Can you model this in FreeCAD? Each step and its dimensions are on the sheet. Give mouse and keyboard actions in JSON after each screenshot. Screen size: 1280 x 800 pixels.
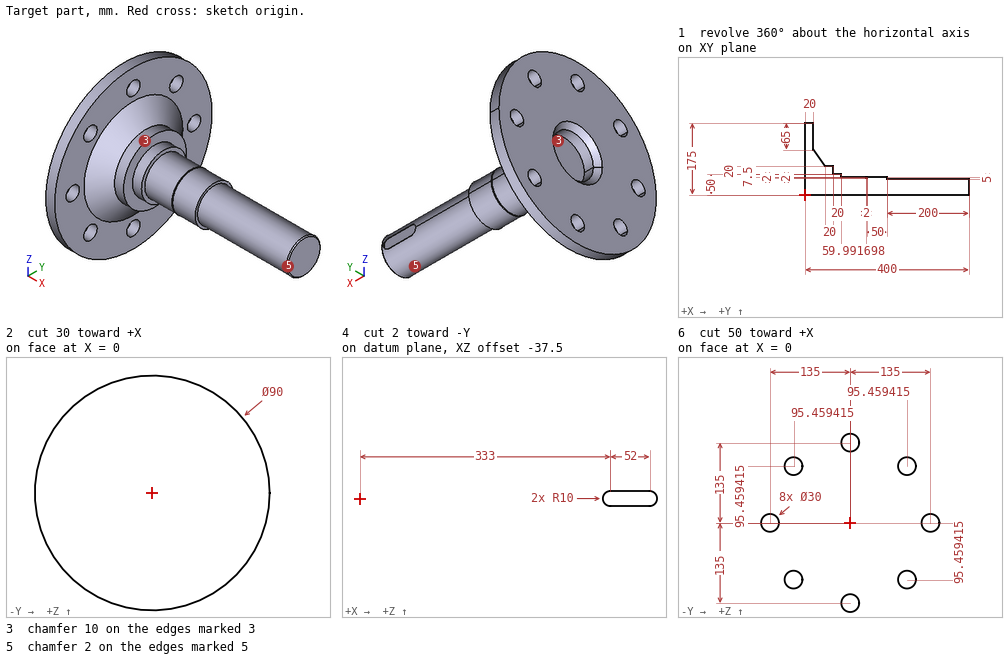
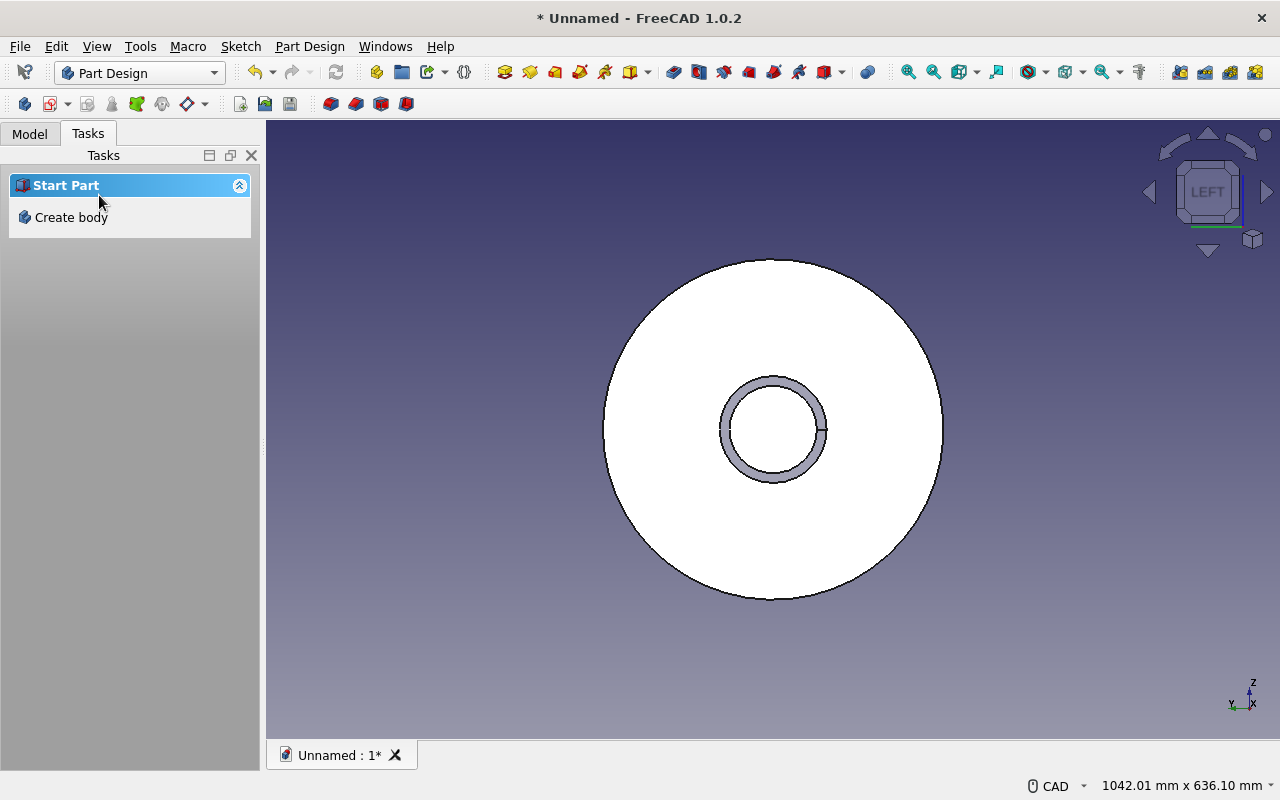
{"action": "left_click", "coordinate": [30, 134]}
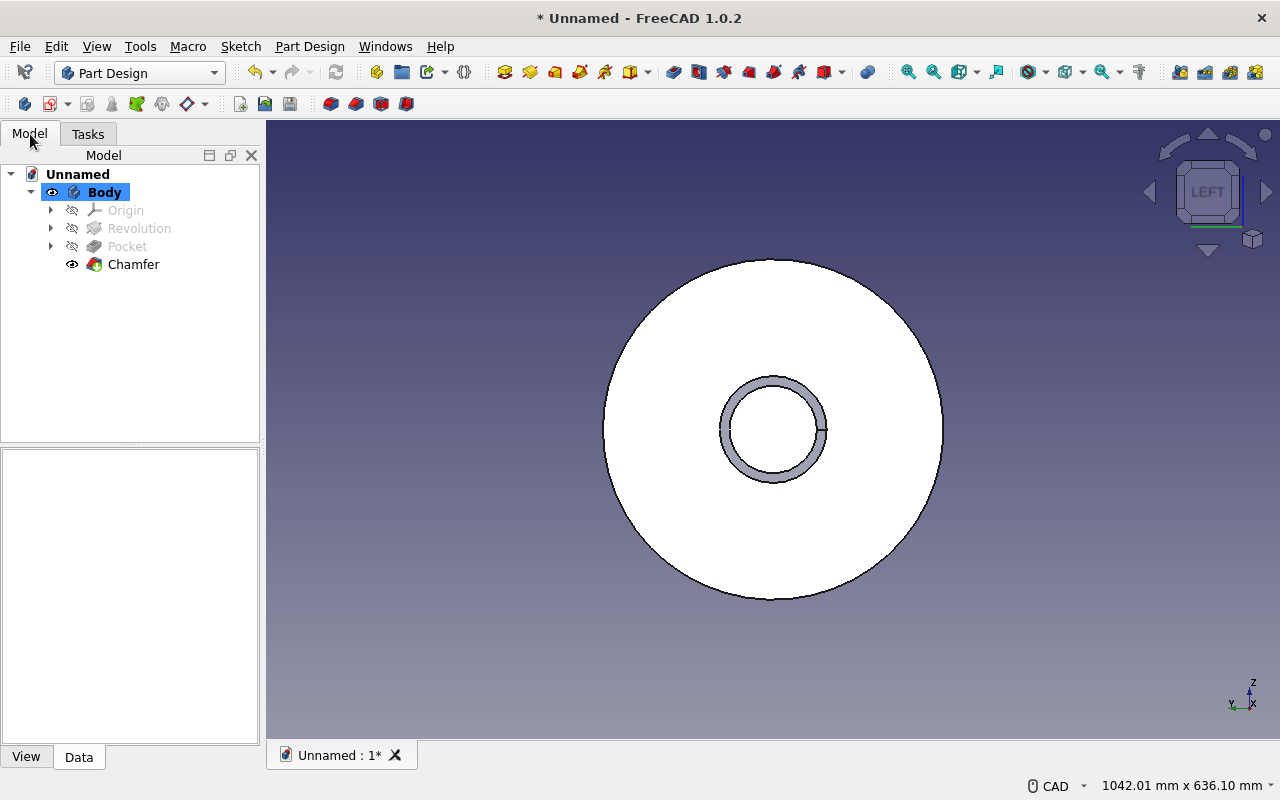
{"action": "left_click", "coordinate": [51, 210]}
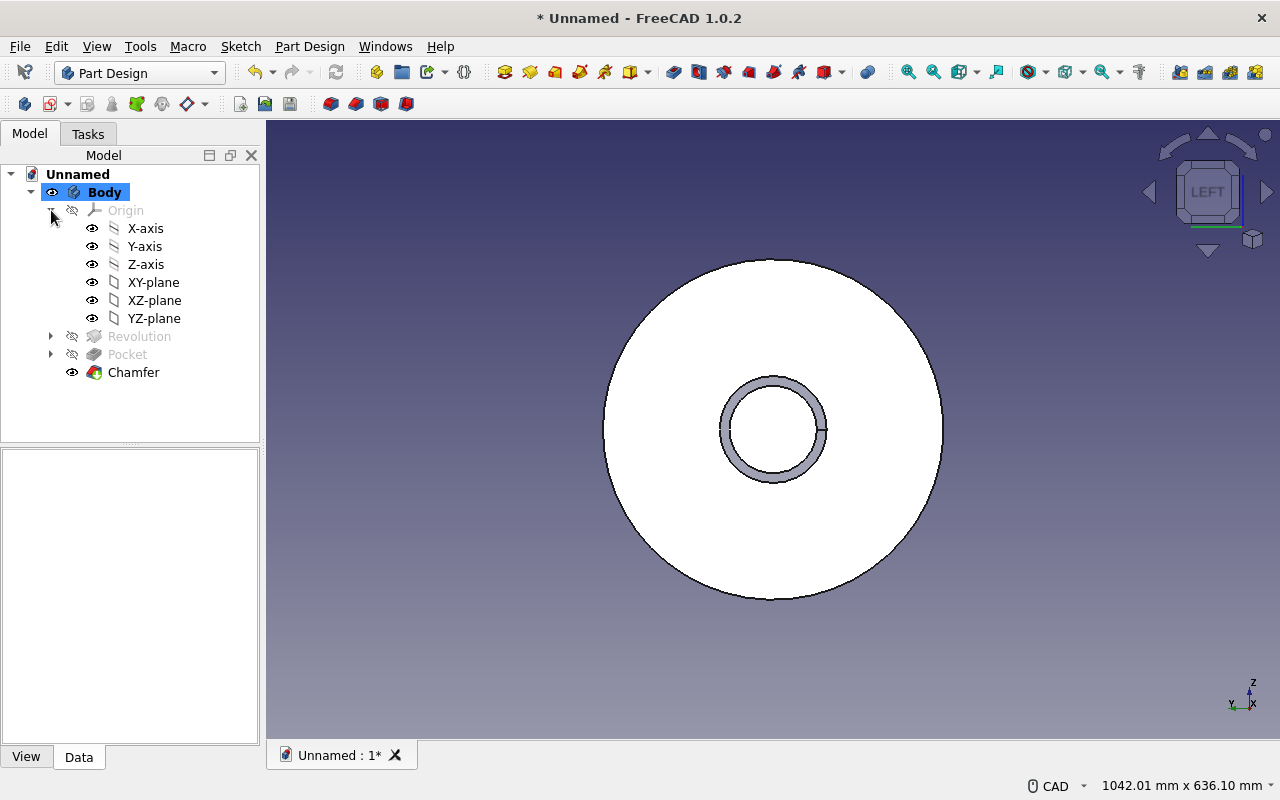
{"action": "left_click", "coordinate": [137, 300]}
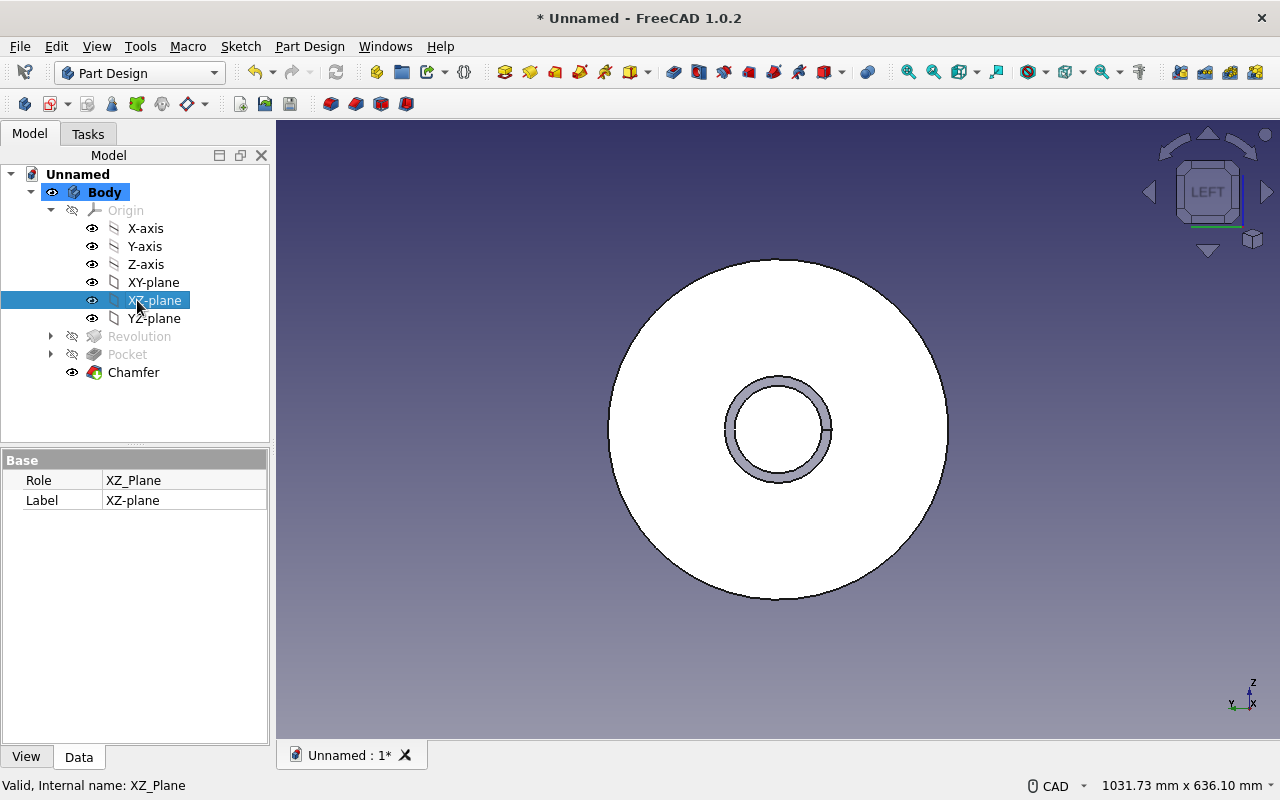
{"action": "left_click", "coordinate": [186, 104]}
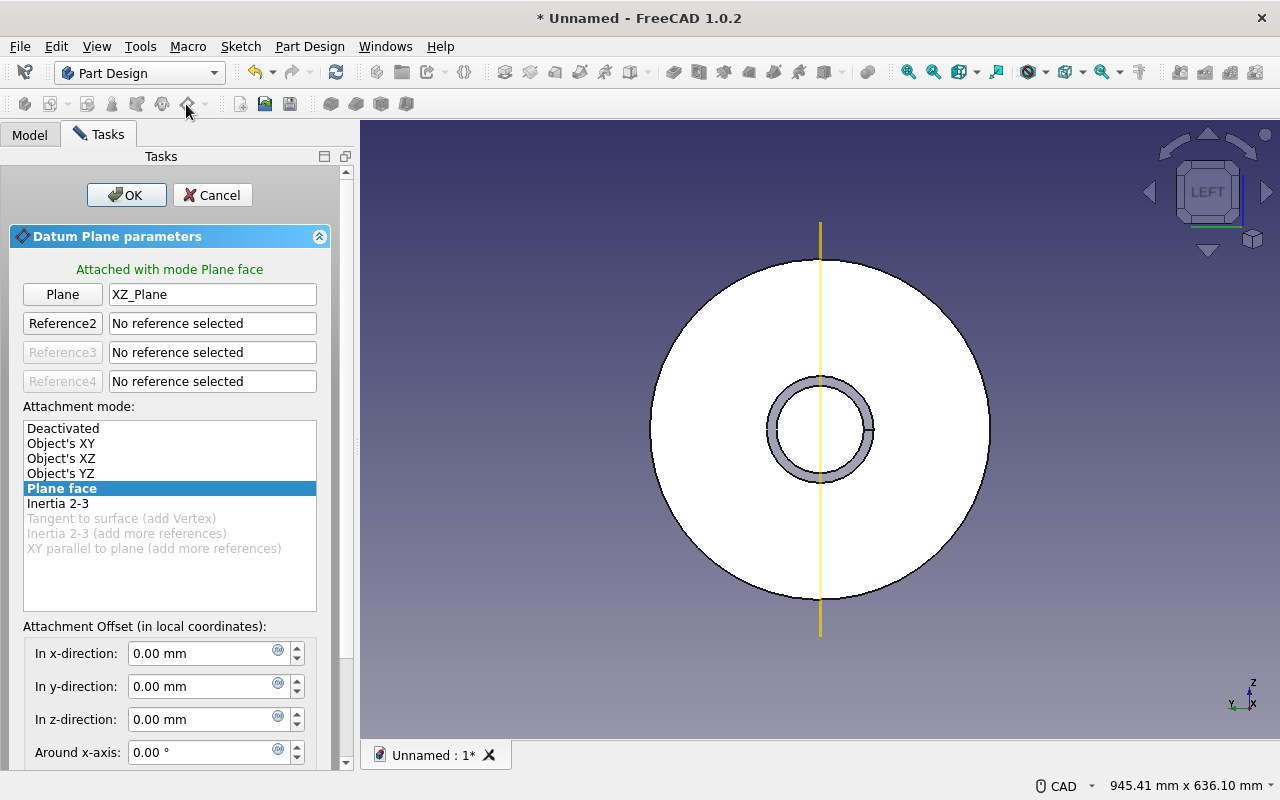
{"action": "triple_click", "coordinate": [210, 720]}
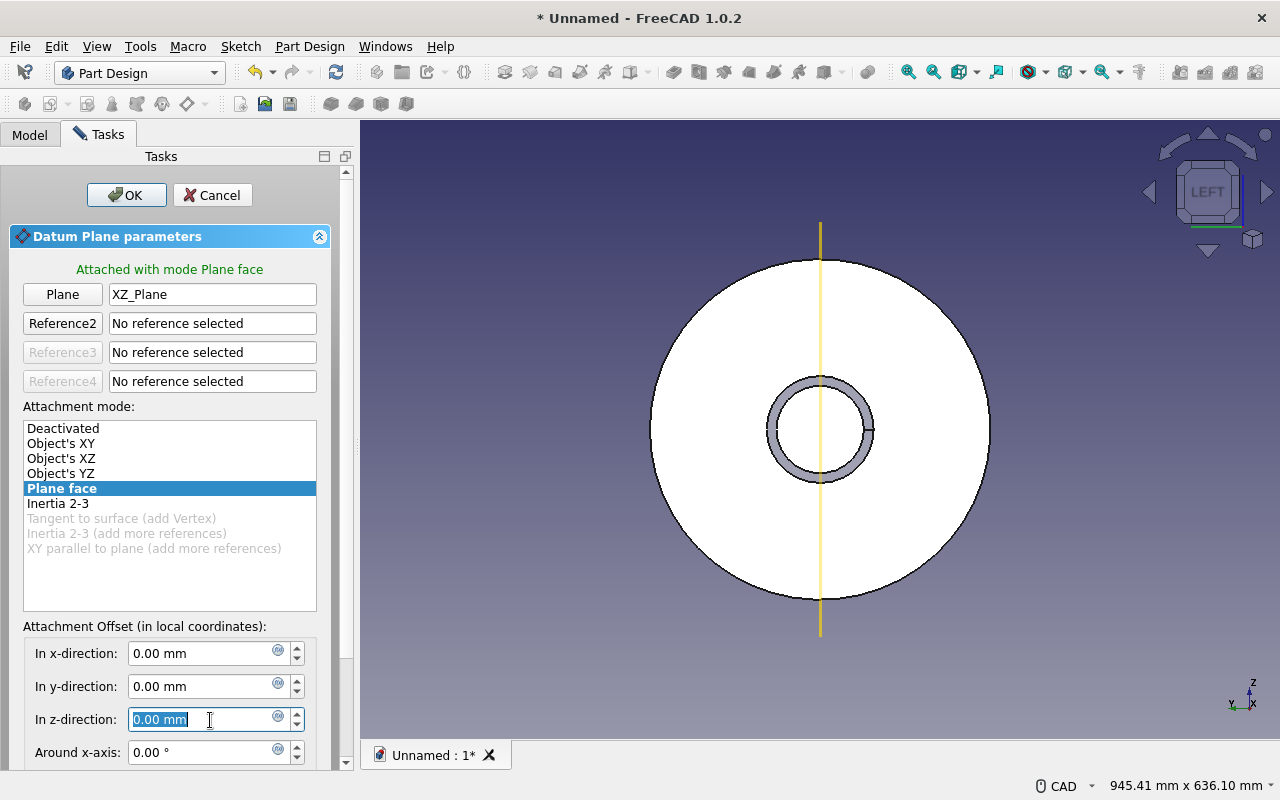
{"action": "type", "text": "-37.5"}
{"action": "key", "text": "Tab"}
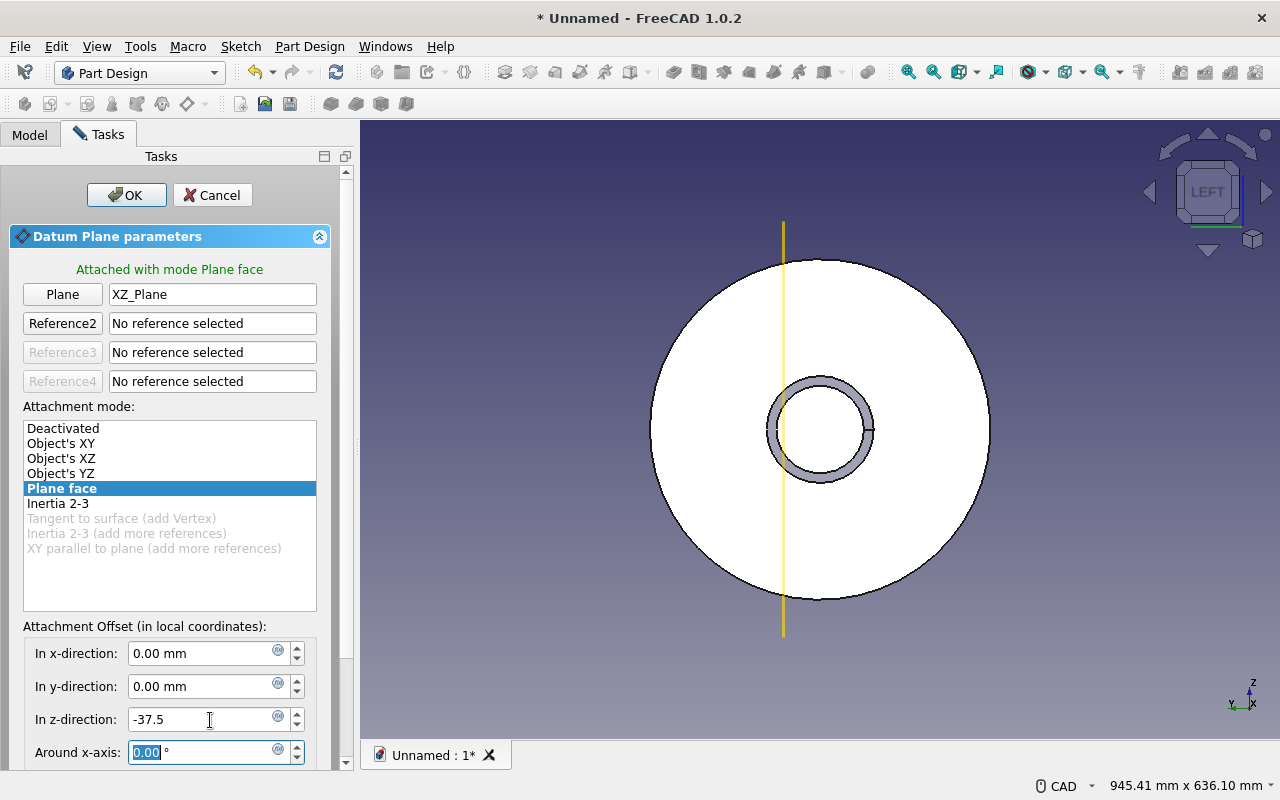
{"action": "left_click", "coordinate": [127, 195]}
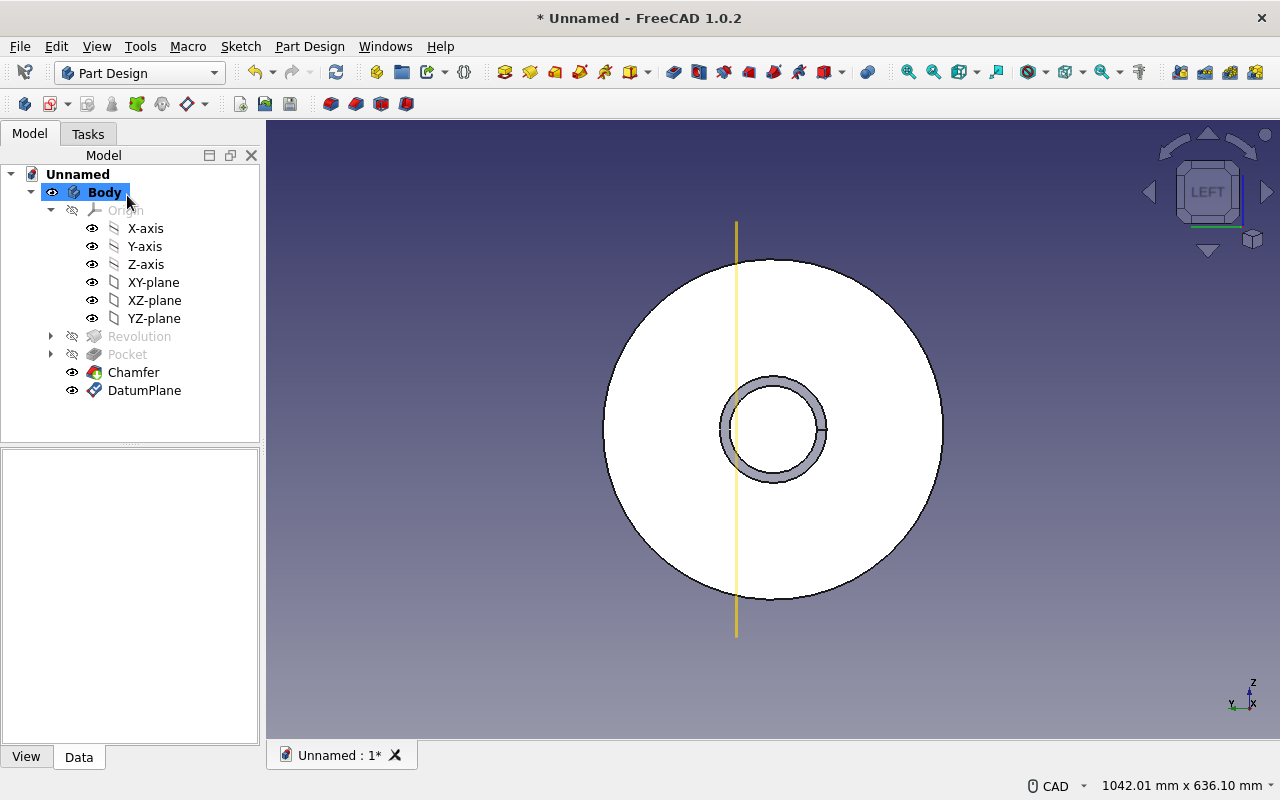
{"action": "left_click", "coordinate": [117, 390]}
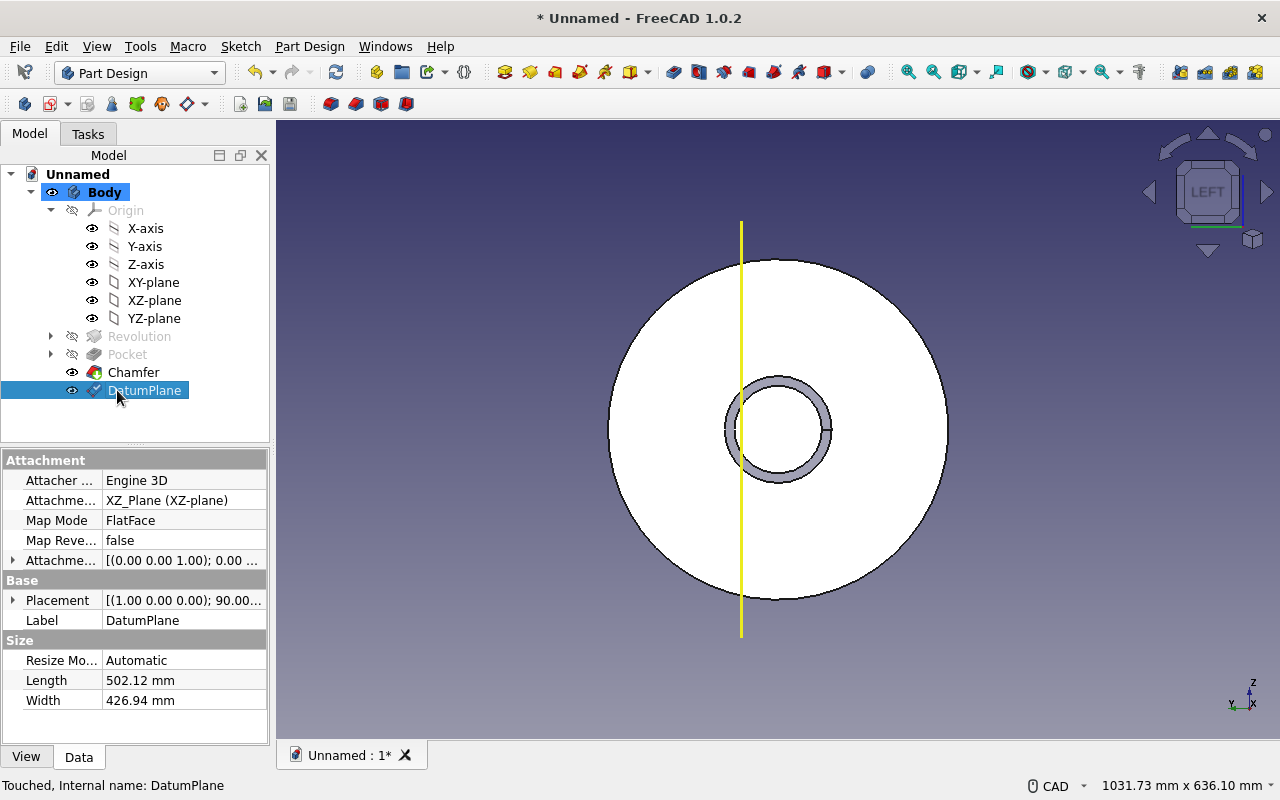
{"action": "left_click", "coordinate": [50, 104]}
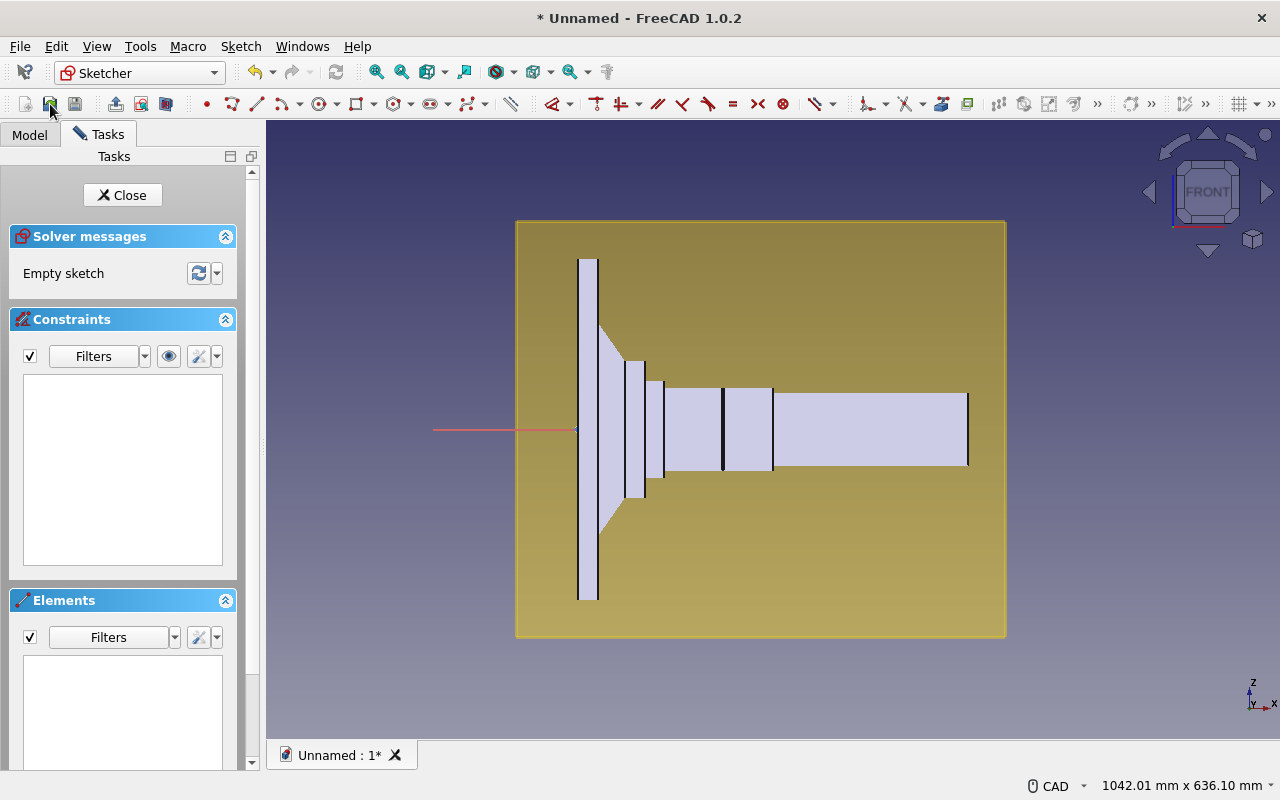
{"action": "left_click", "coordinate": [166, 104]}